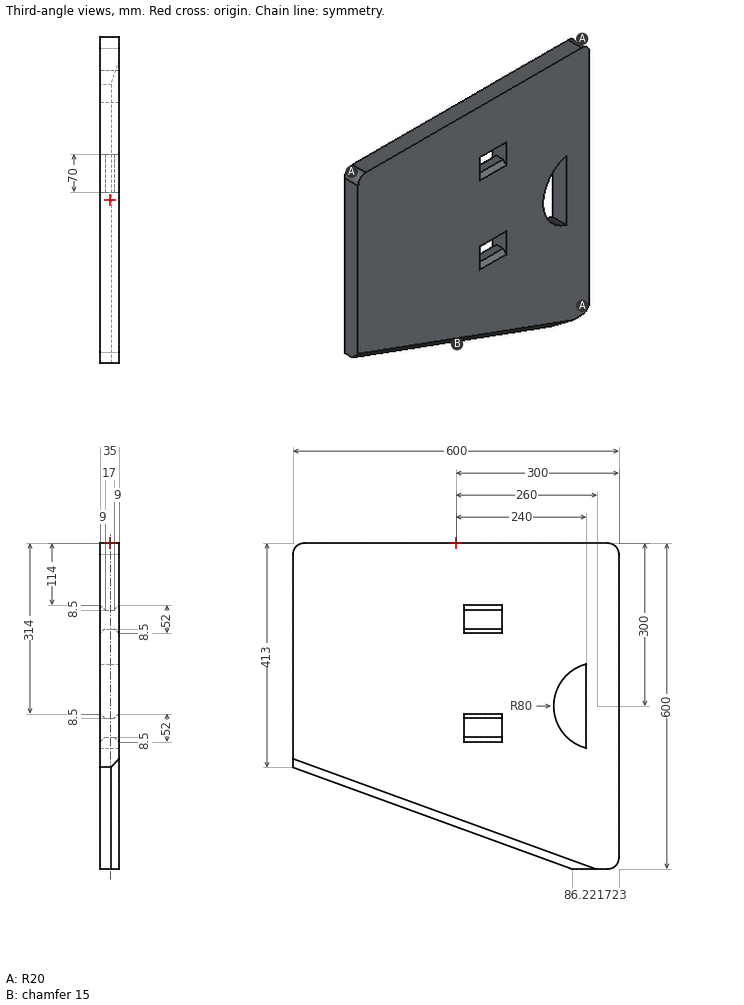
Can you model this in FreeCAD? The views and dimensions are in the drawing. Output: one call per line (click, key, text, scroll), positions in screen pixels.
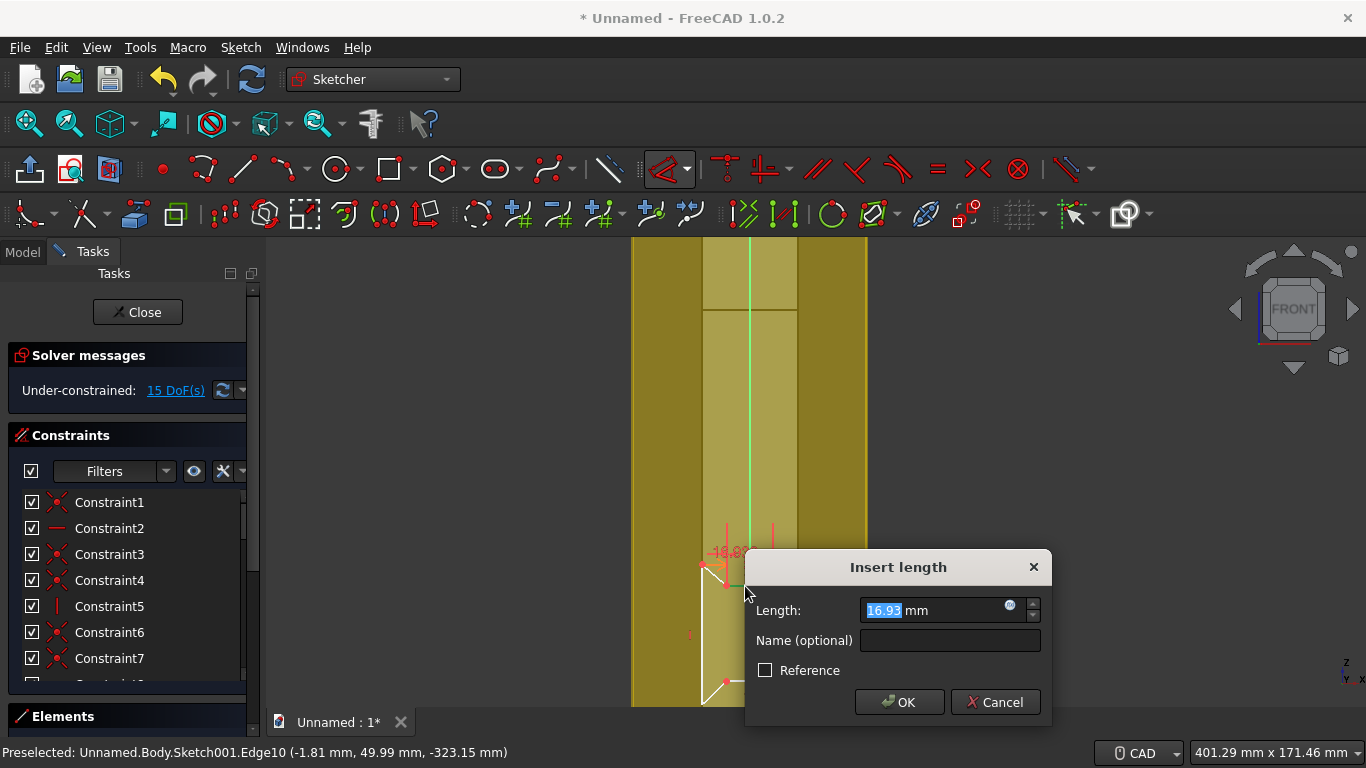
text(17)
key(Return)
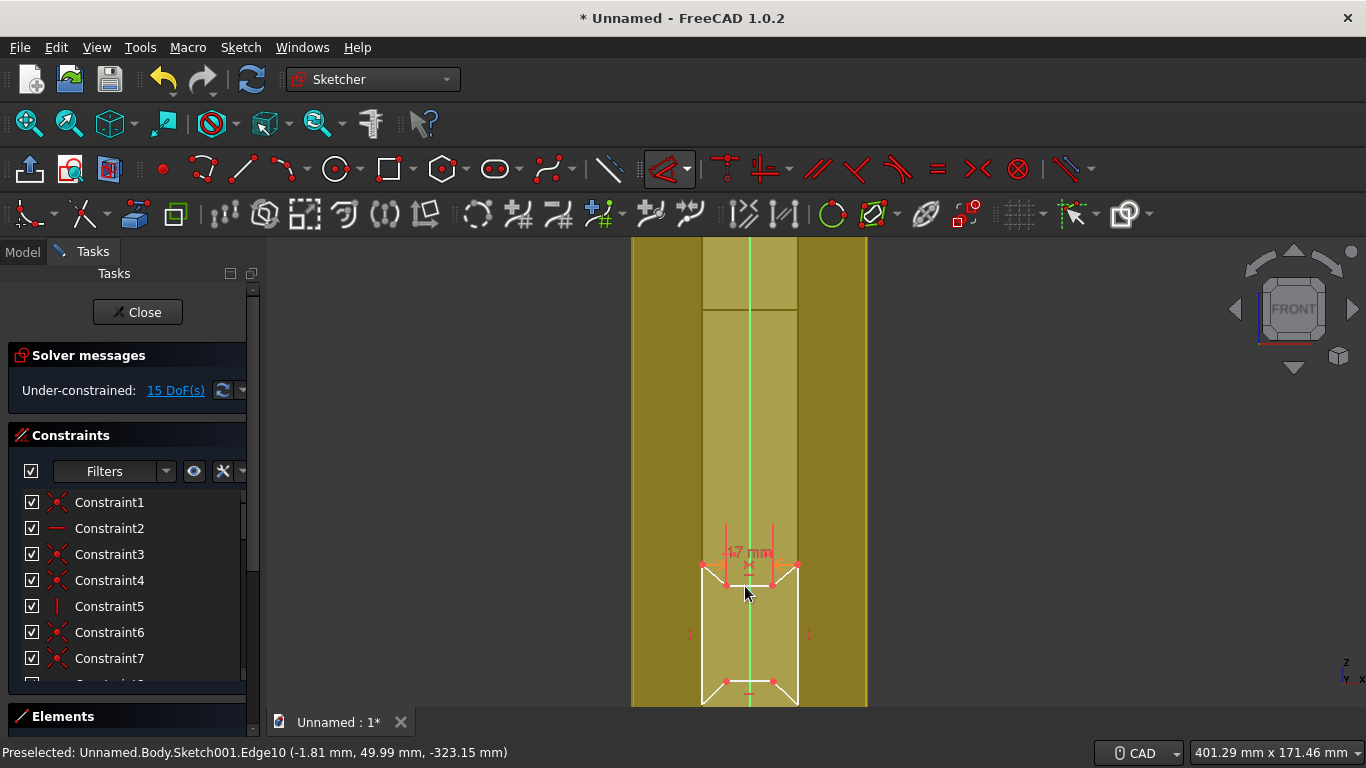
click(798, 607)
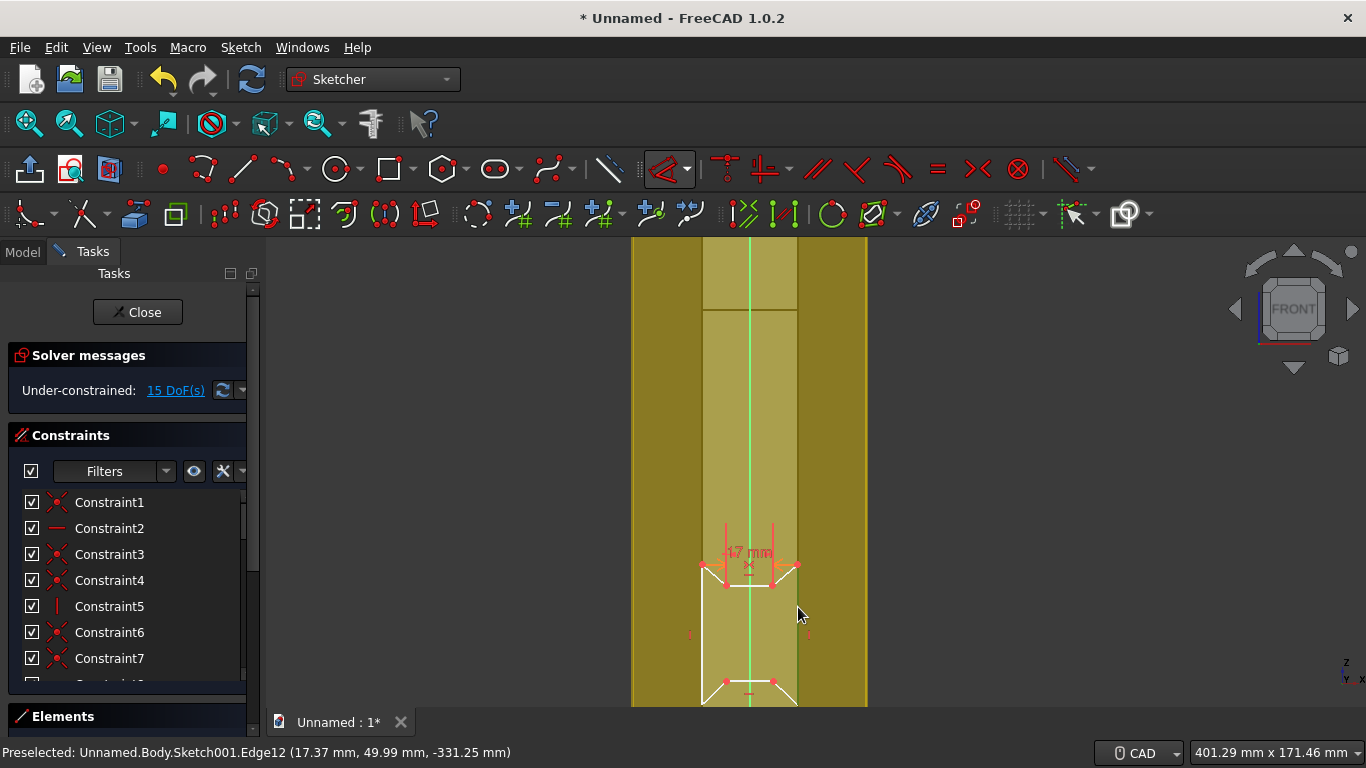
click(690, 170)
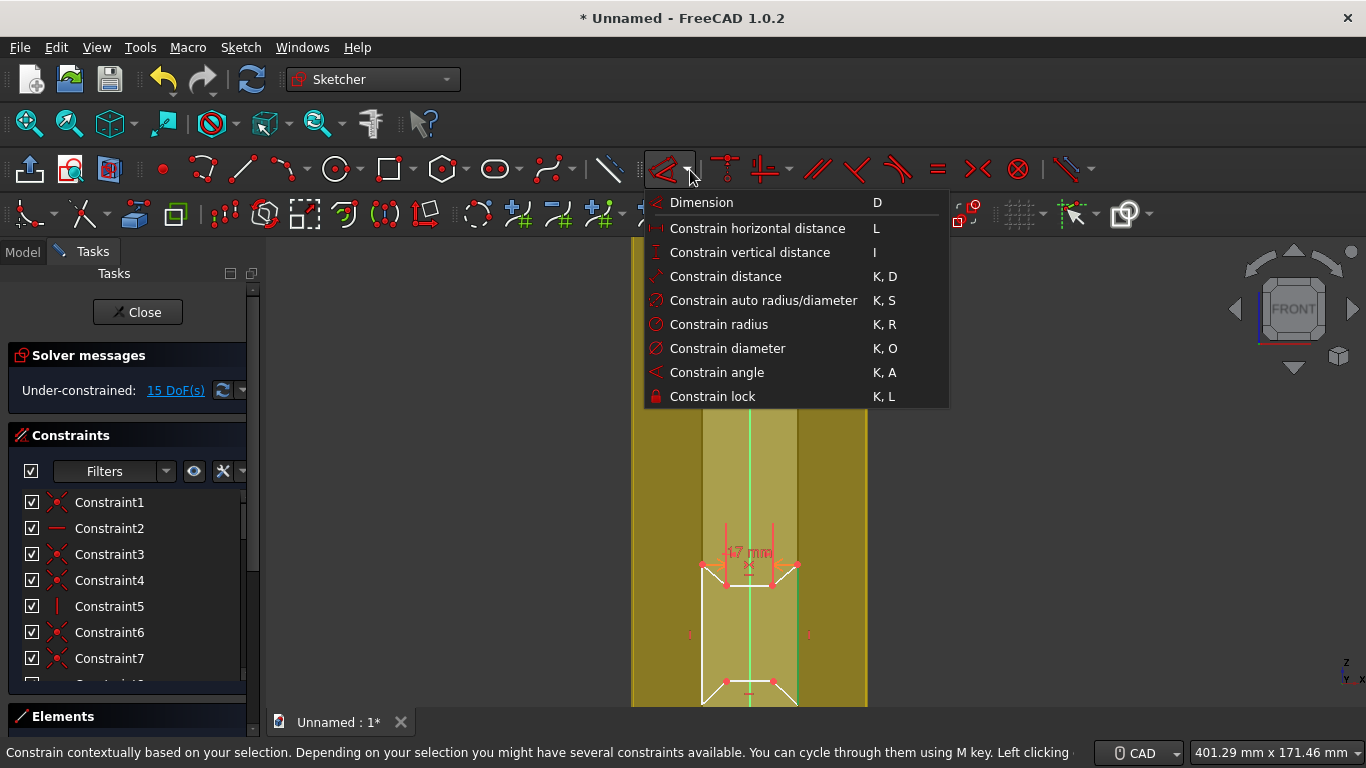
click(797, 252)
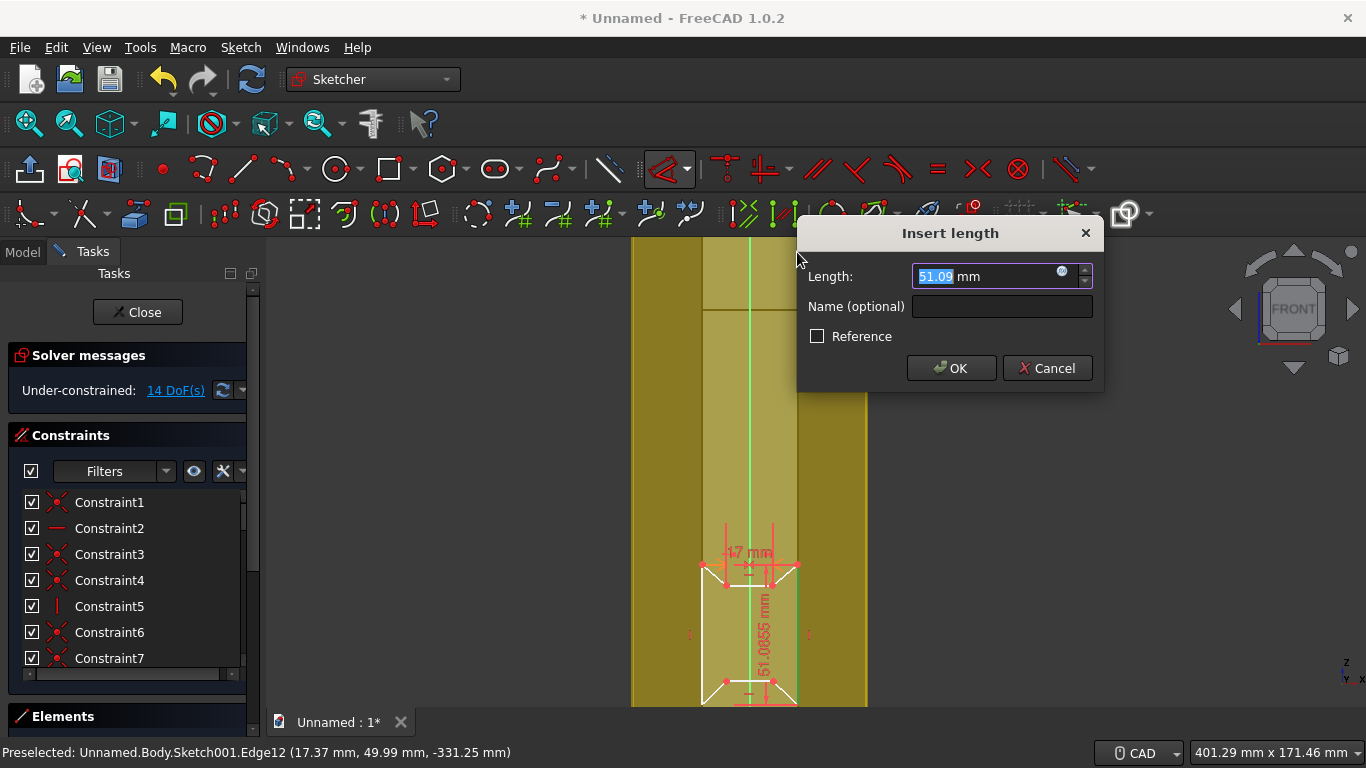
text(52)
key(Return)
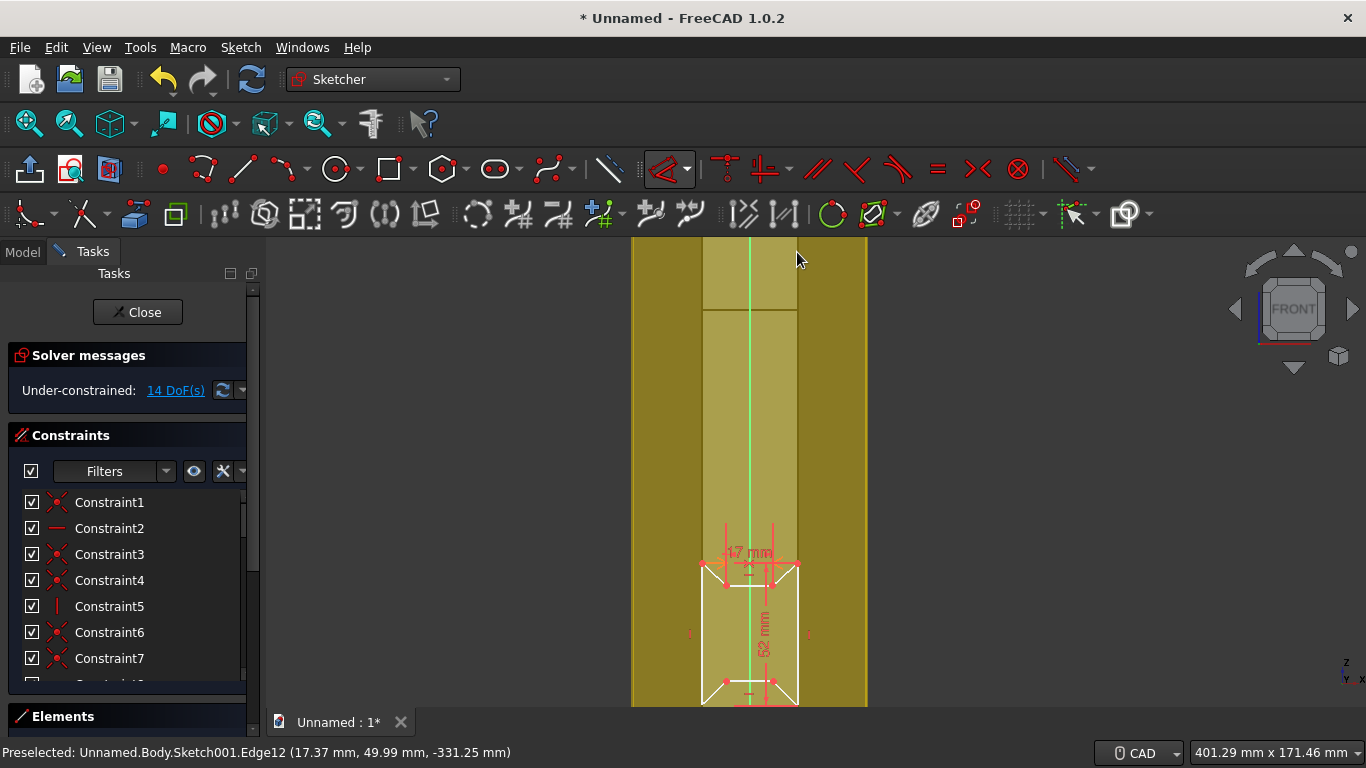
scroll(746, 589, down, 6)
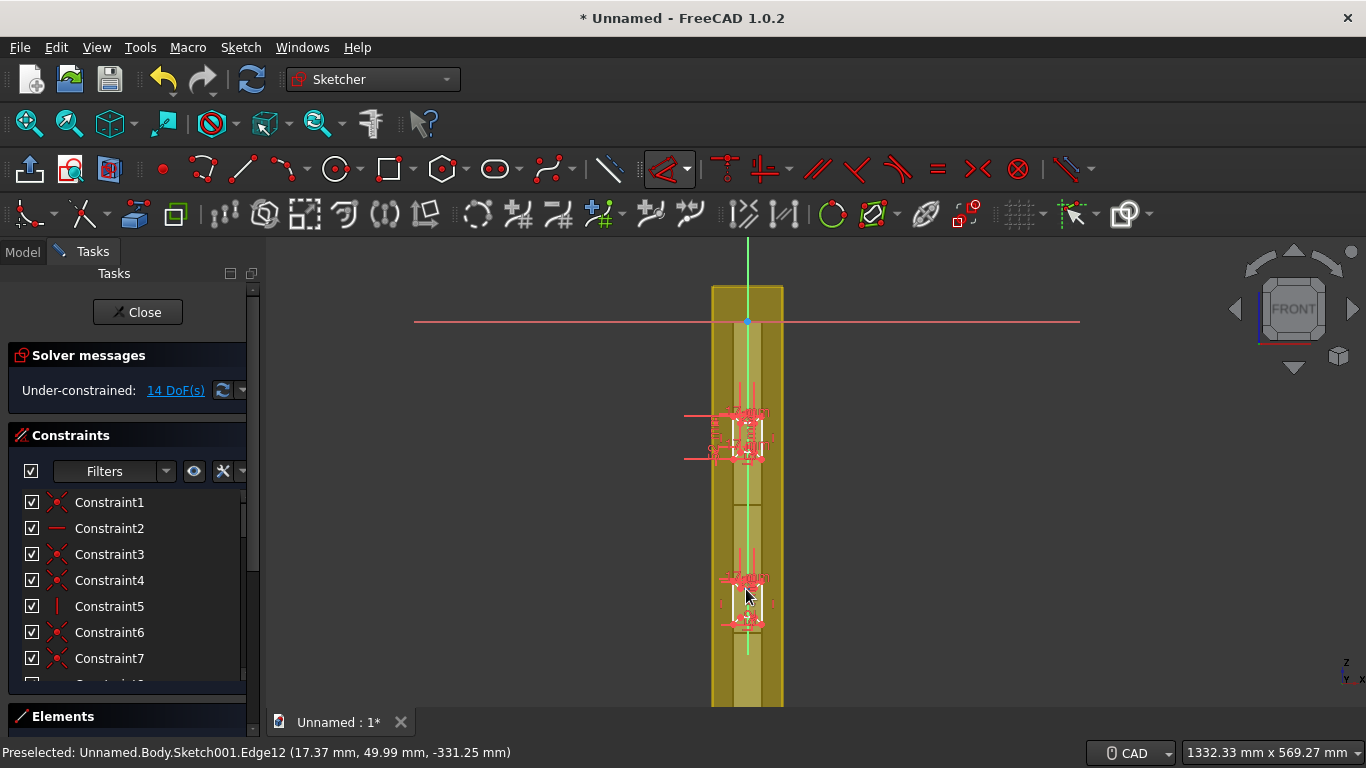
scroll(750, 617, up, 9)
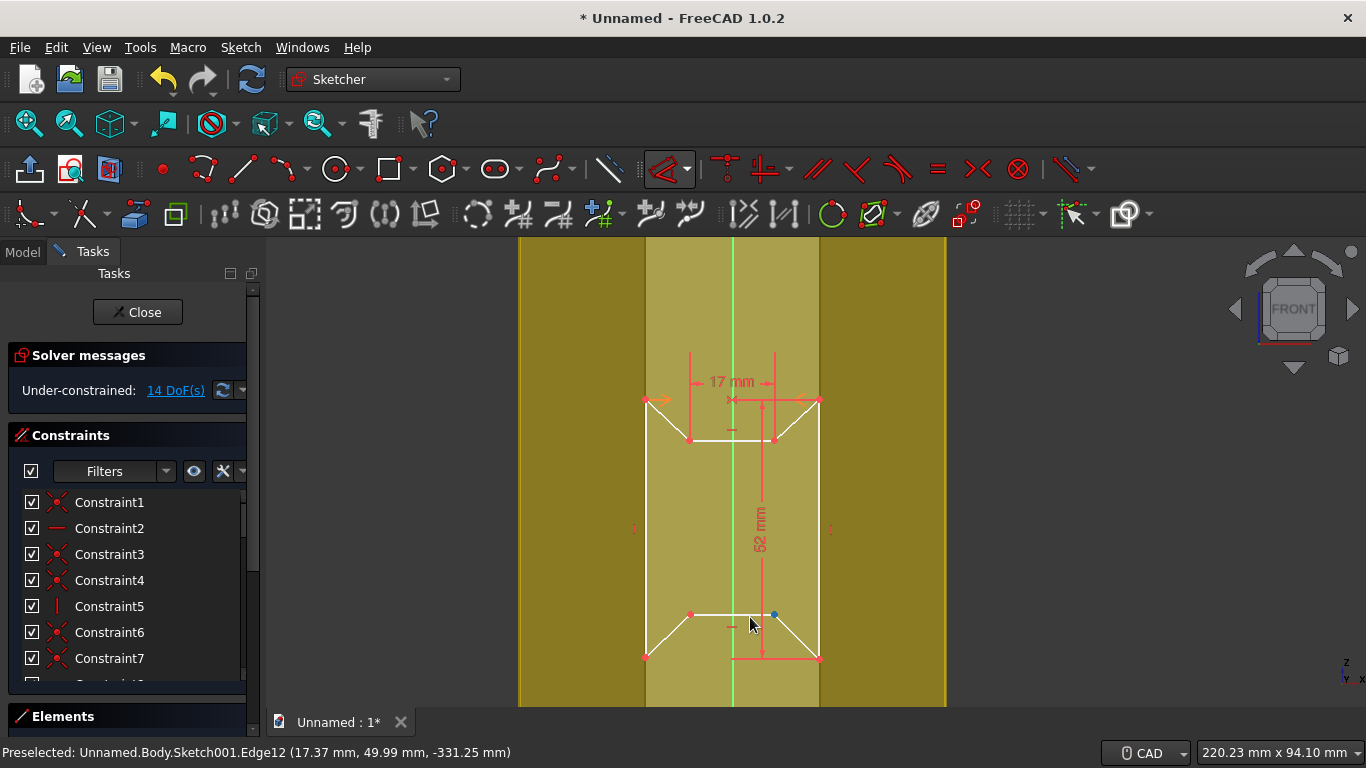
click(749, 615)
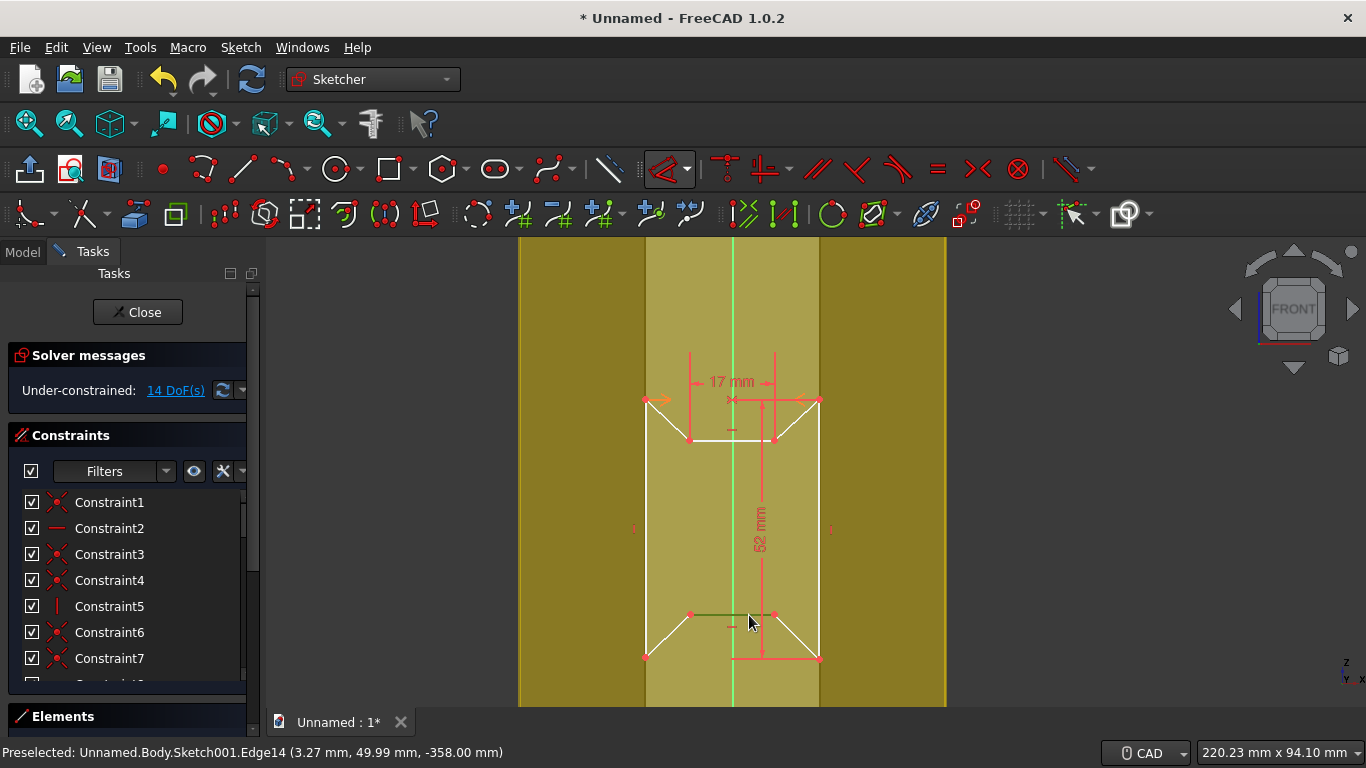
click(690, 170)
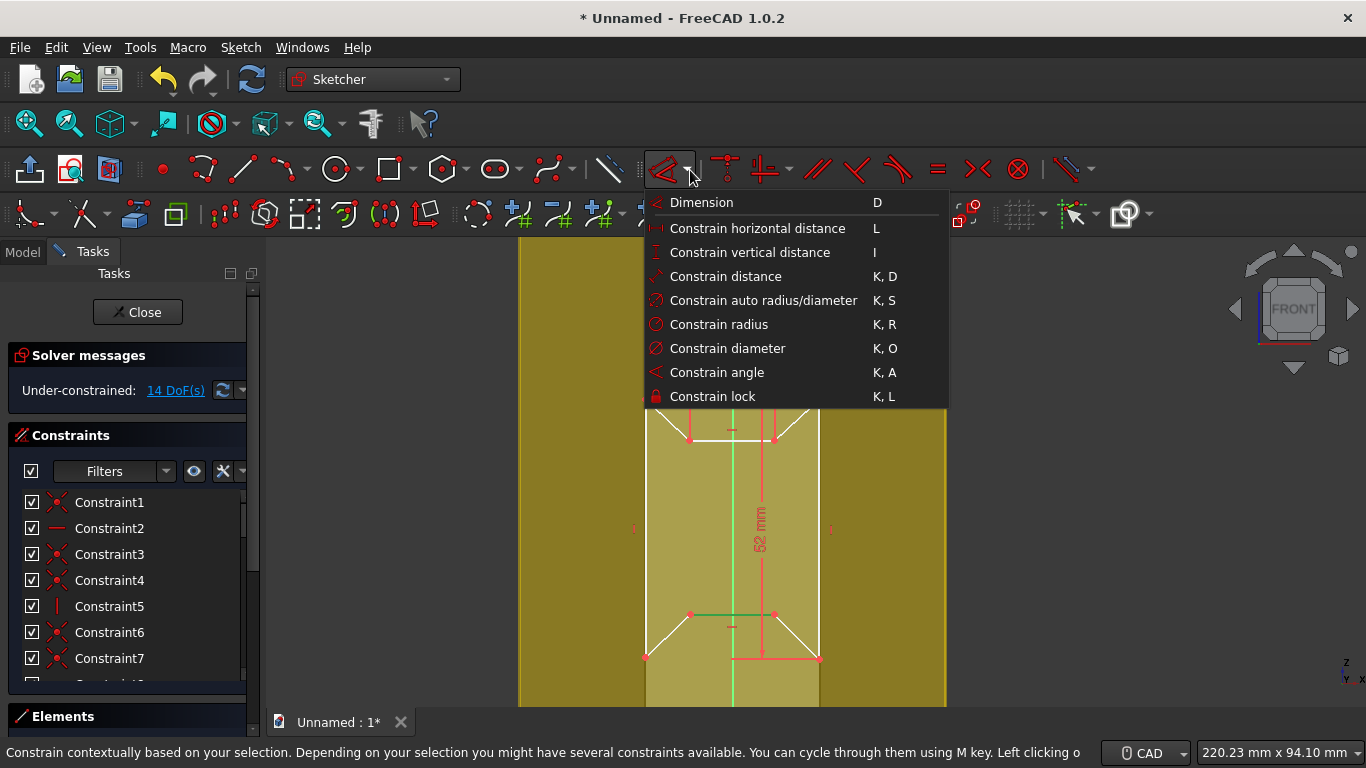
click(797, 228)